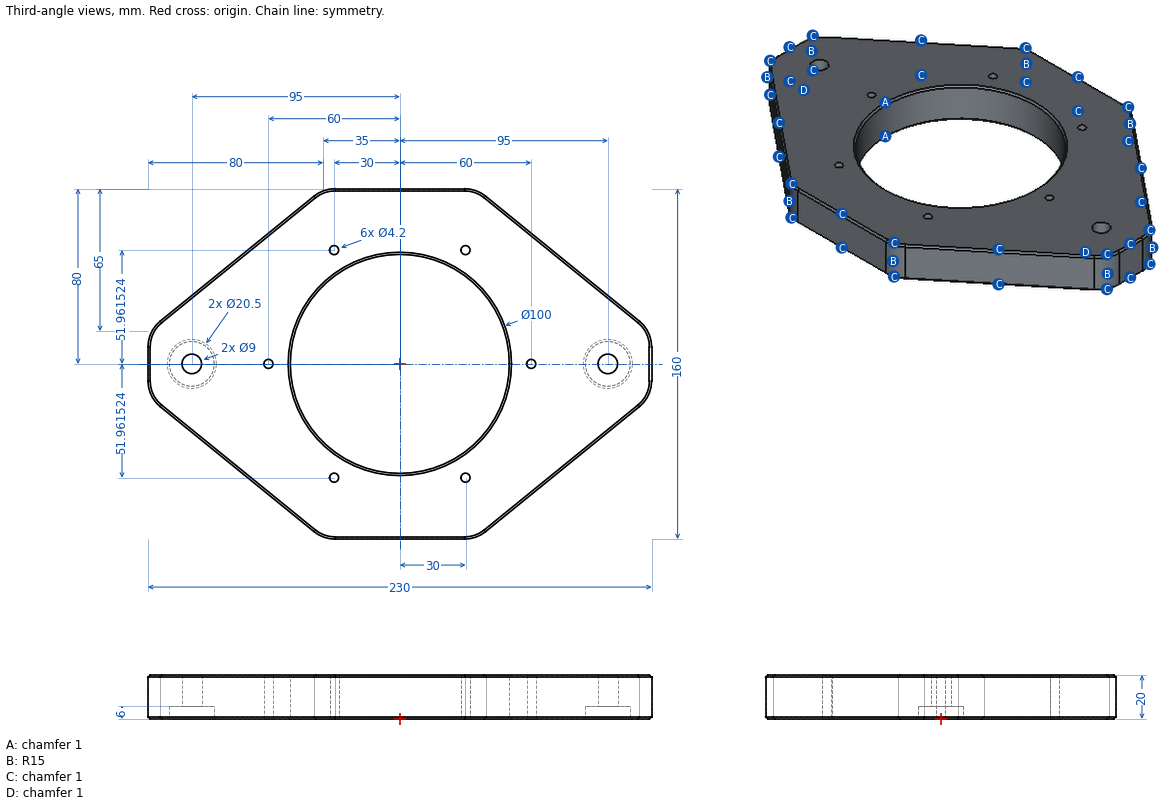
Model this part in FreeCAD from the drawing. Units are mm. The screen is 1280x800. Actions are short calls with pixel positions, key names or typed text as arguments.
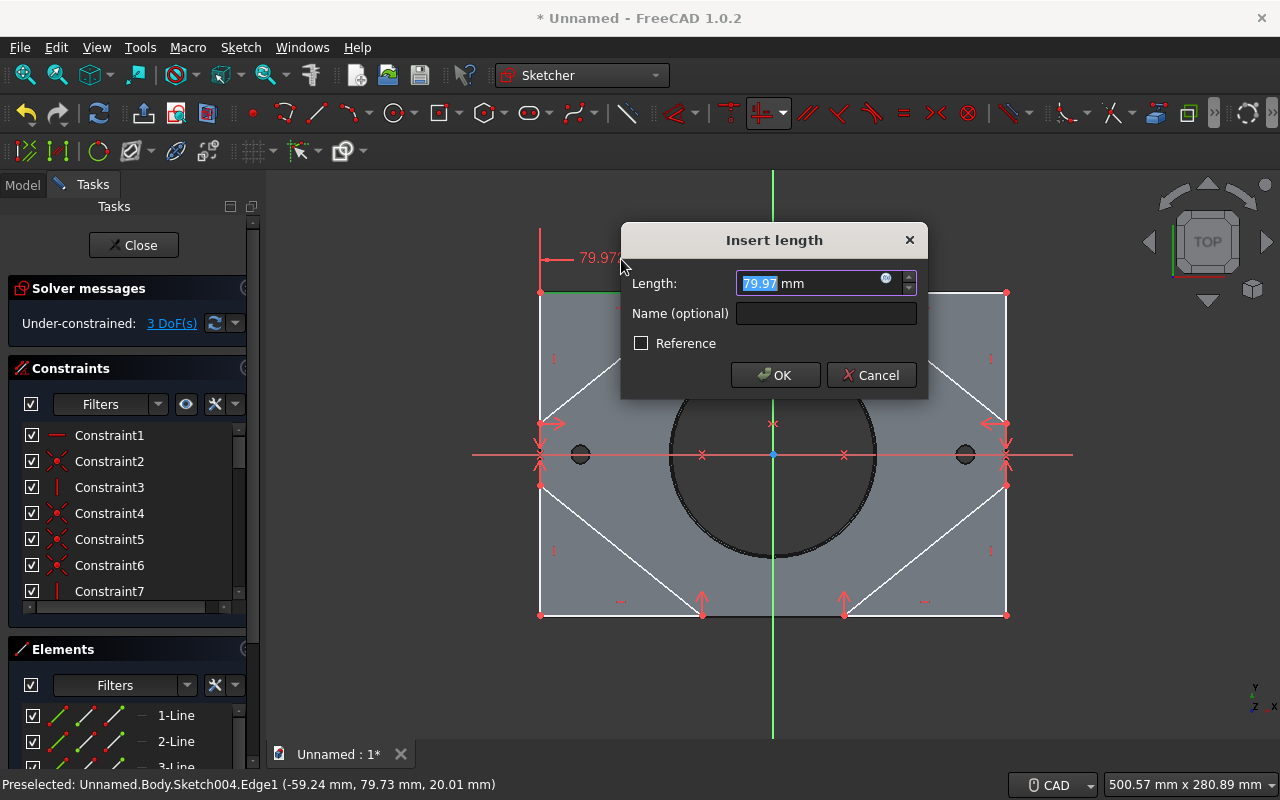
text(80)
key(Return)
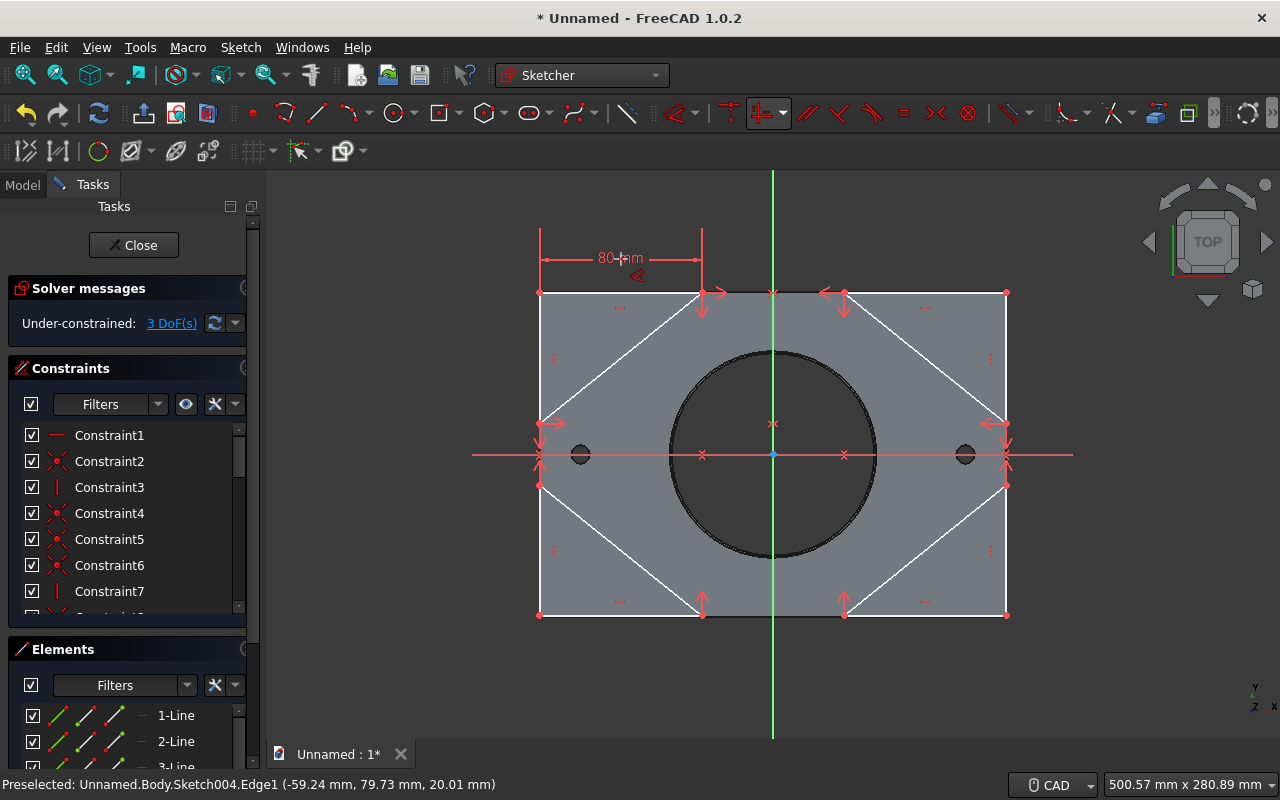
click(540, 332)
click(506, 358)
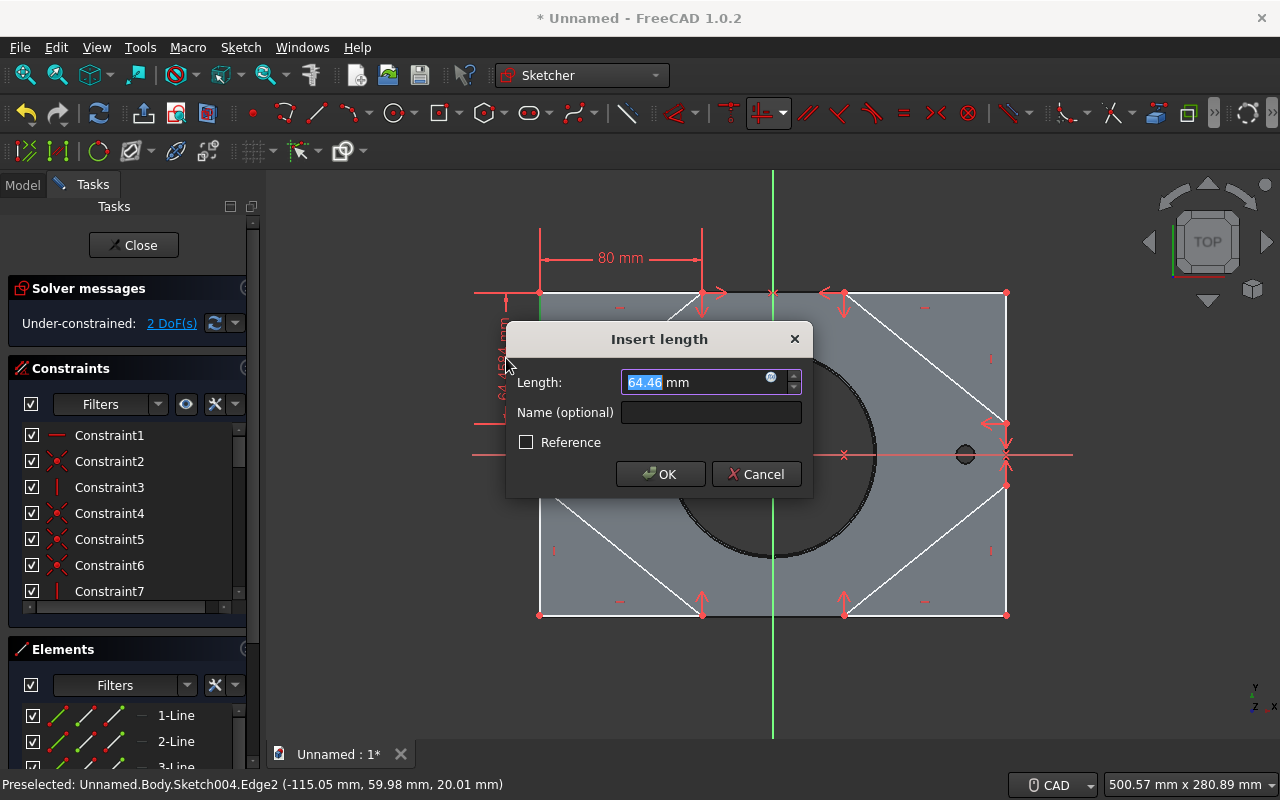
text(65)
key(Return)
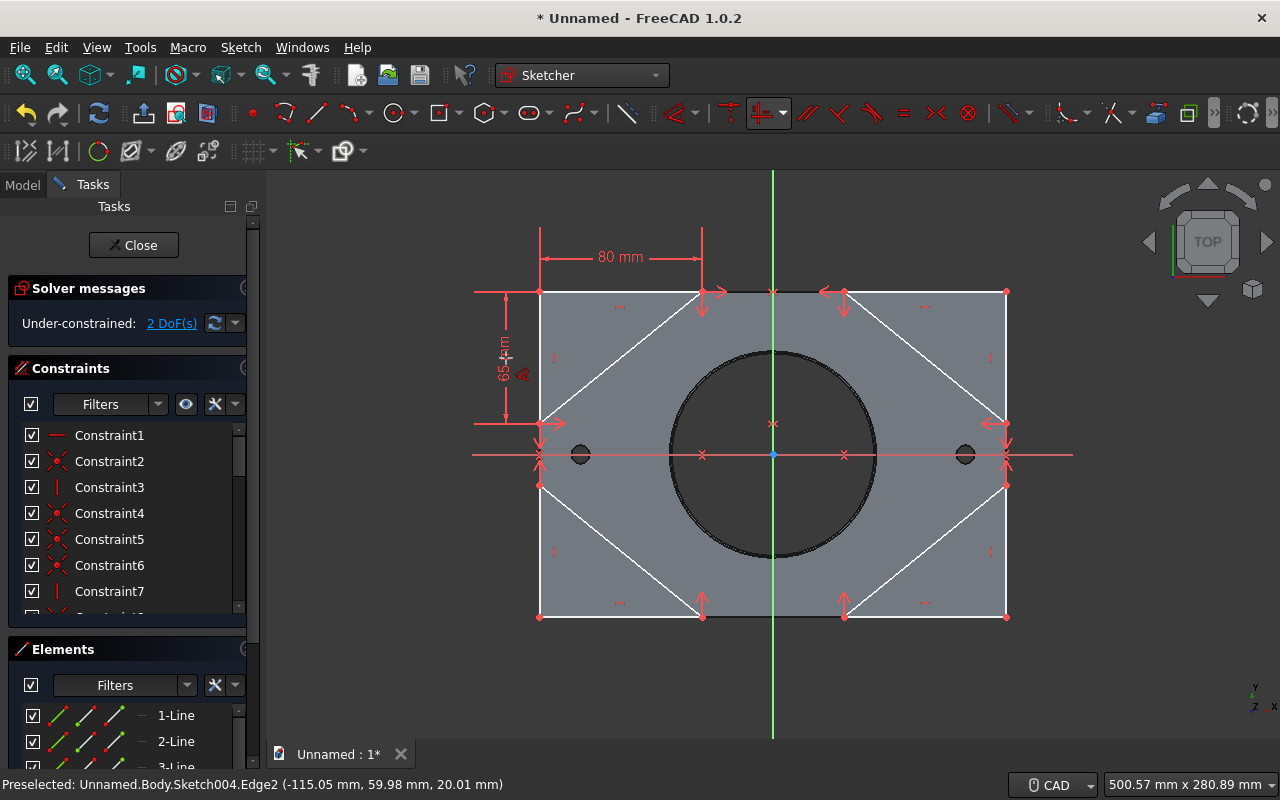
click(702, 292)
click(737, 258)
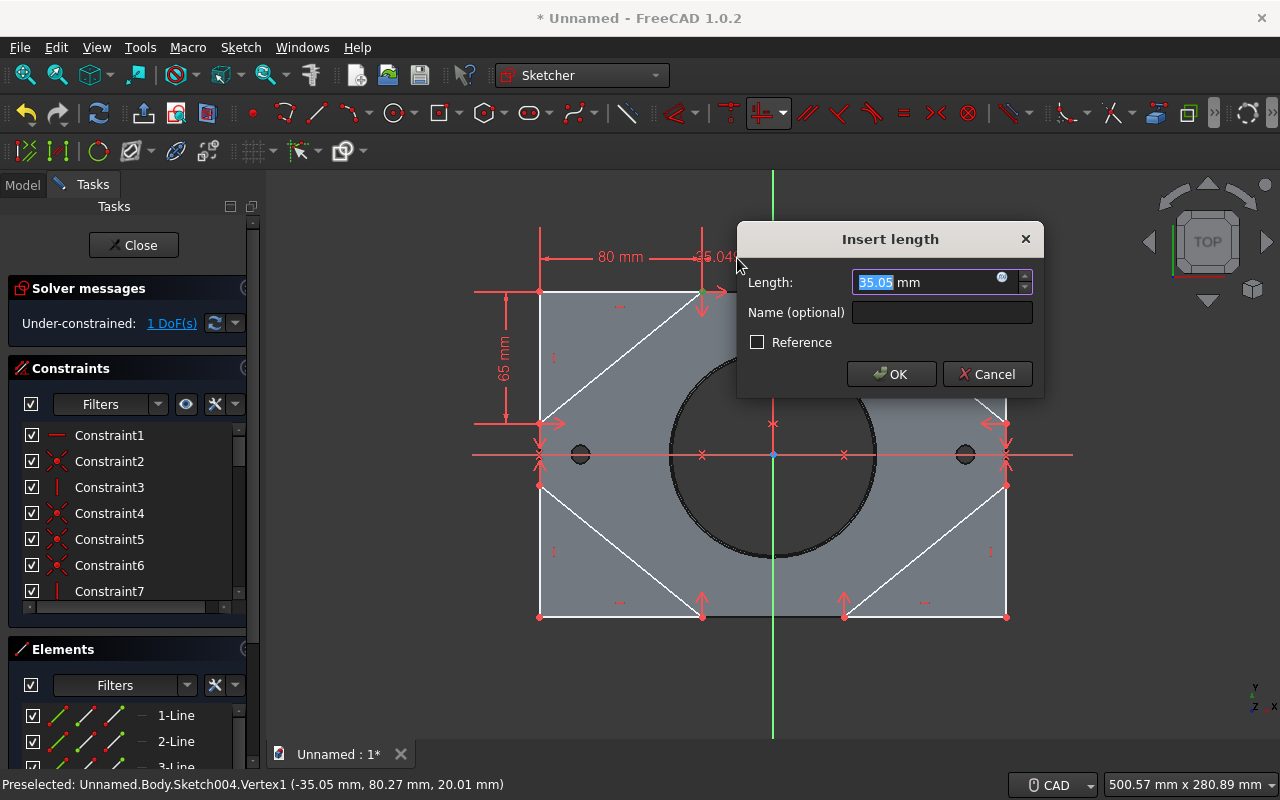
text(35)
key(Return)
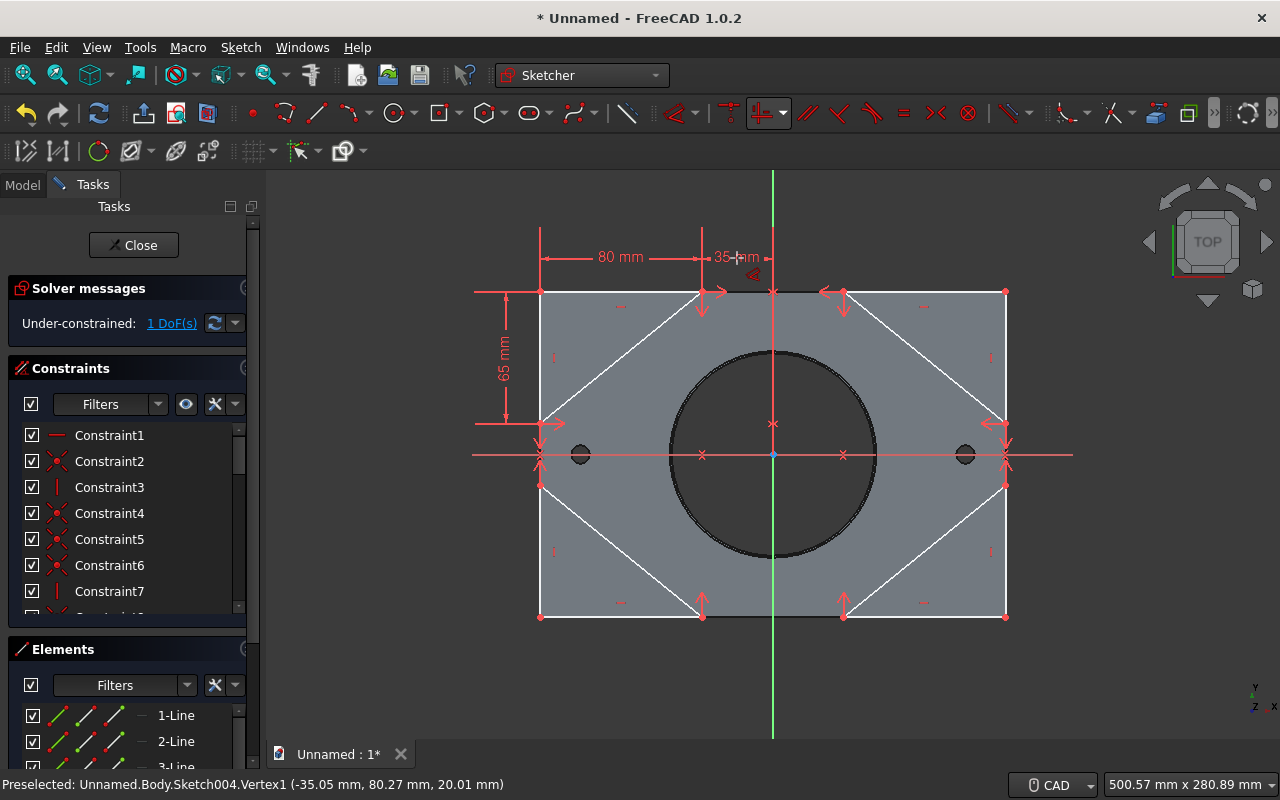
click(702, 292)
click(668, 373)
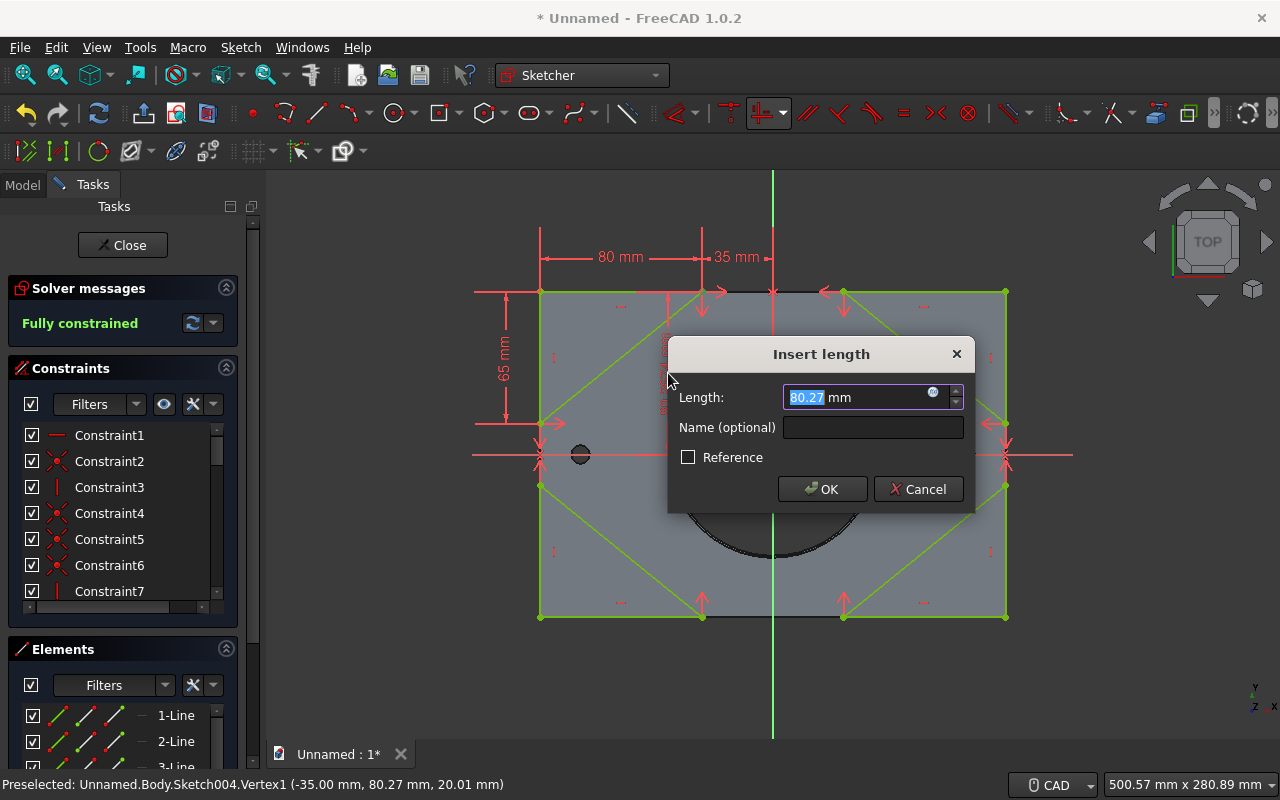
text(80)
key(Return)
key(Escape)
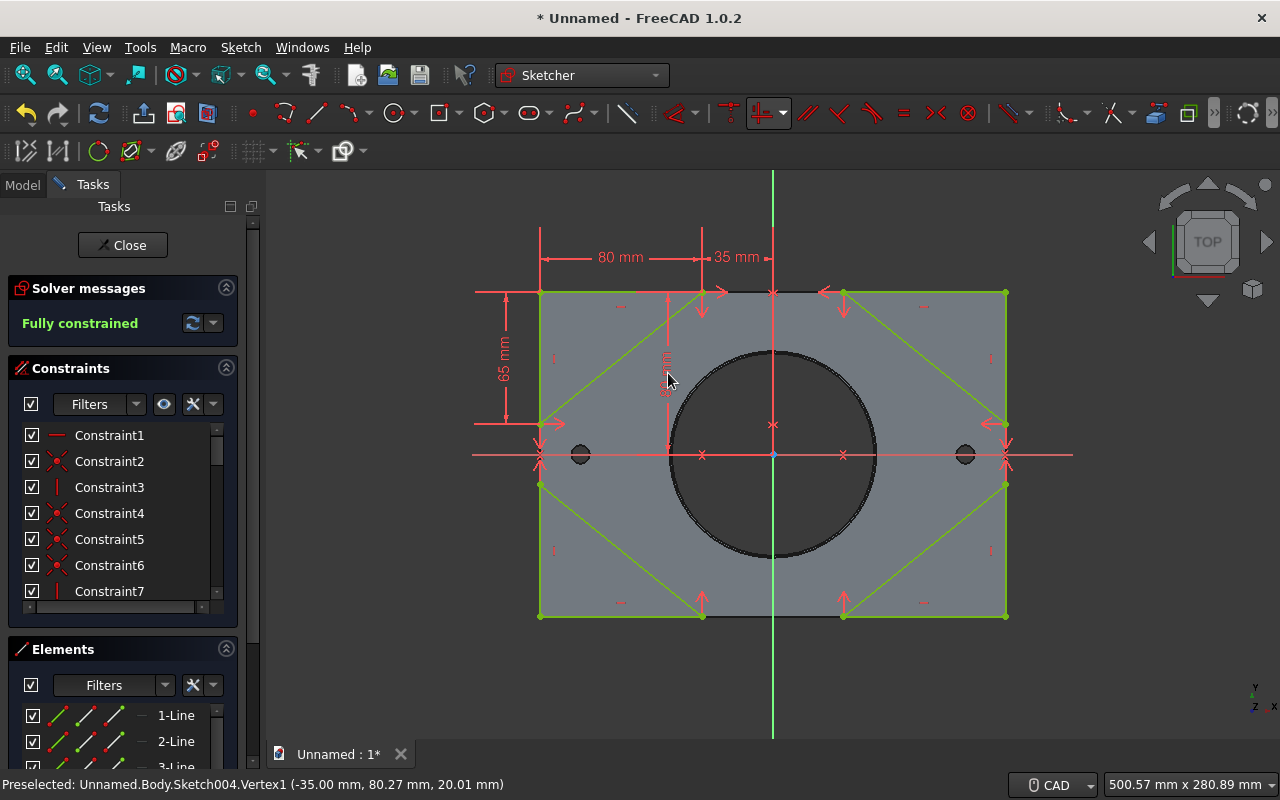
click(123, 245)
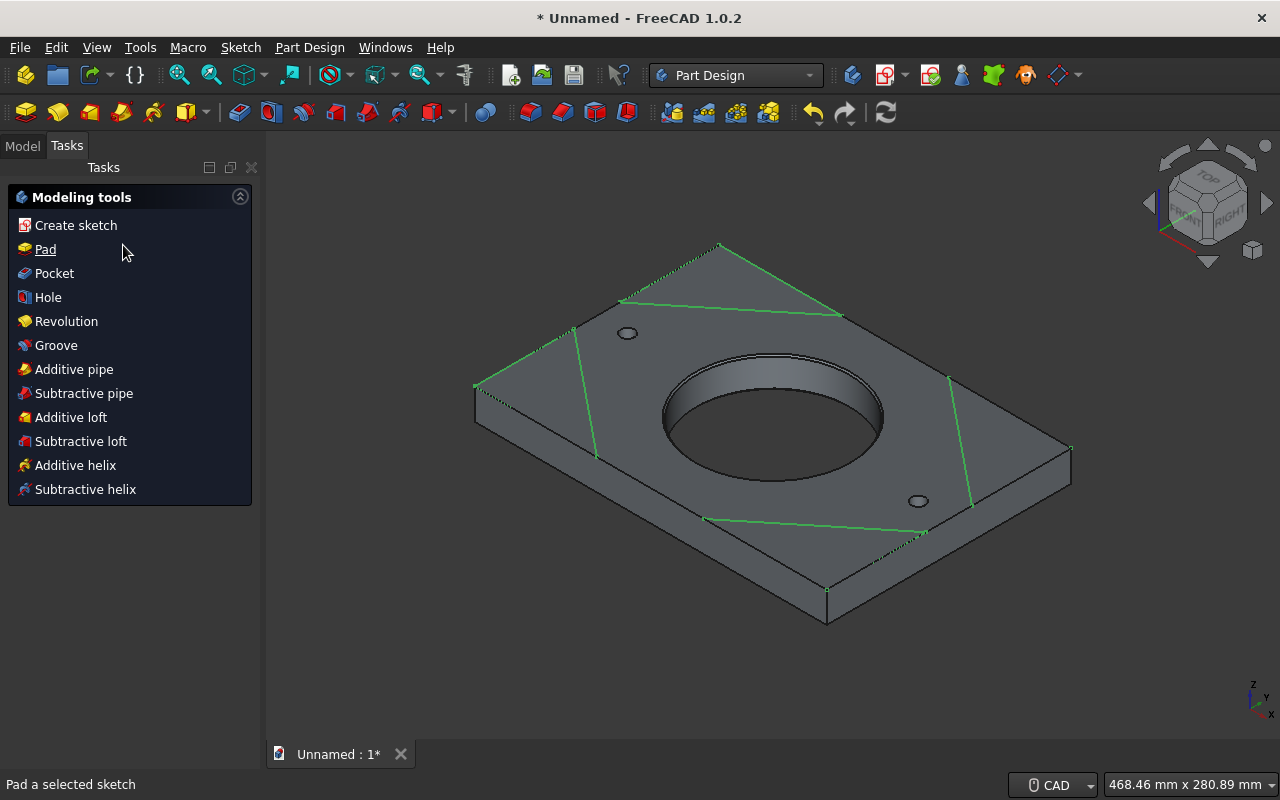
click(240, 112)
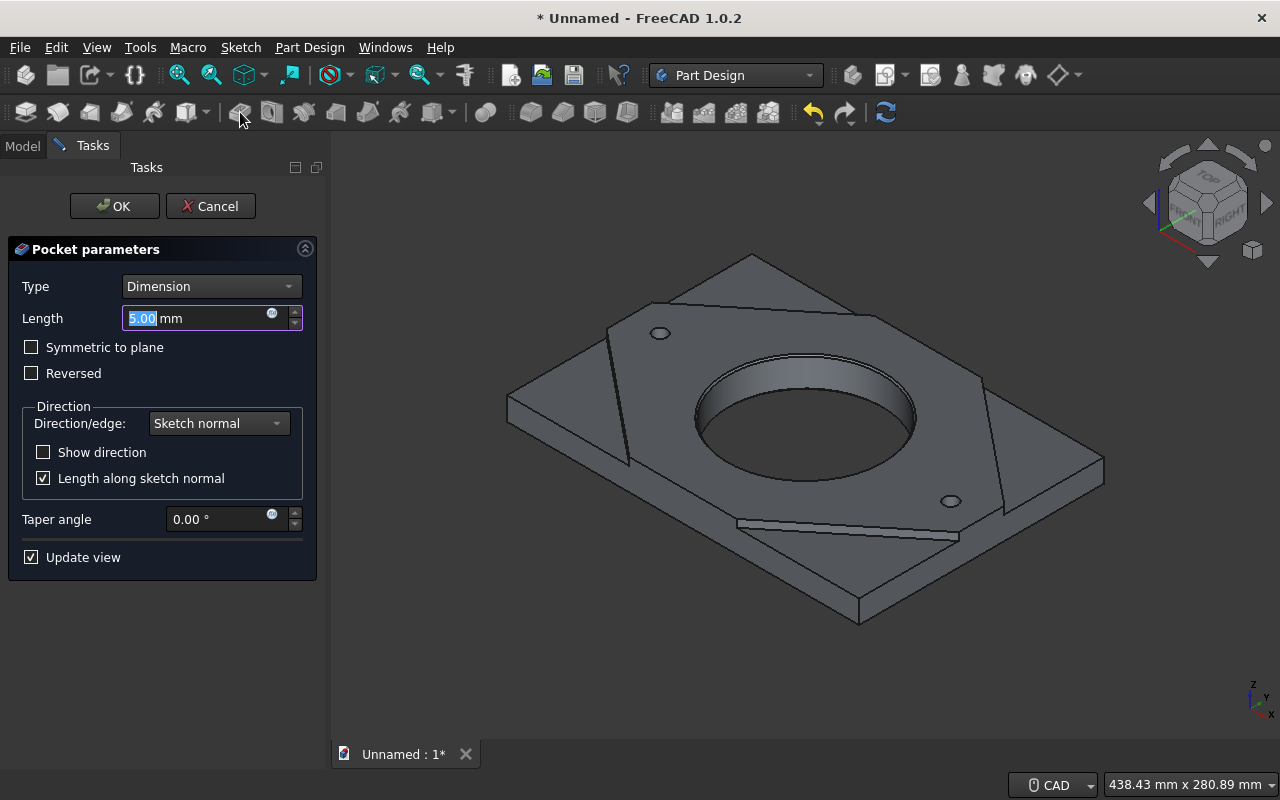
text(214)
key(Tab)